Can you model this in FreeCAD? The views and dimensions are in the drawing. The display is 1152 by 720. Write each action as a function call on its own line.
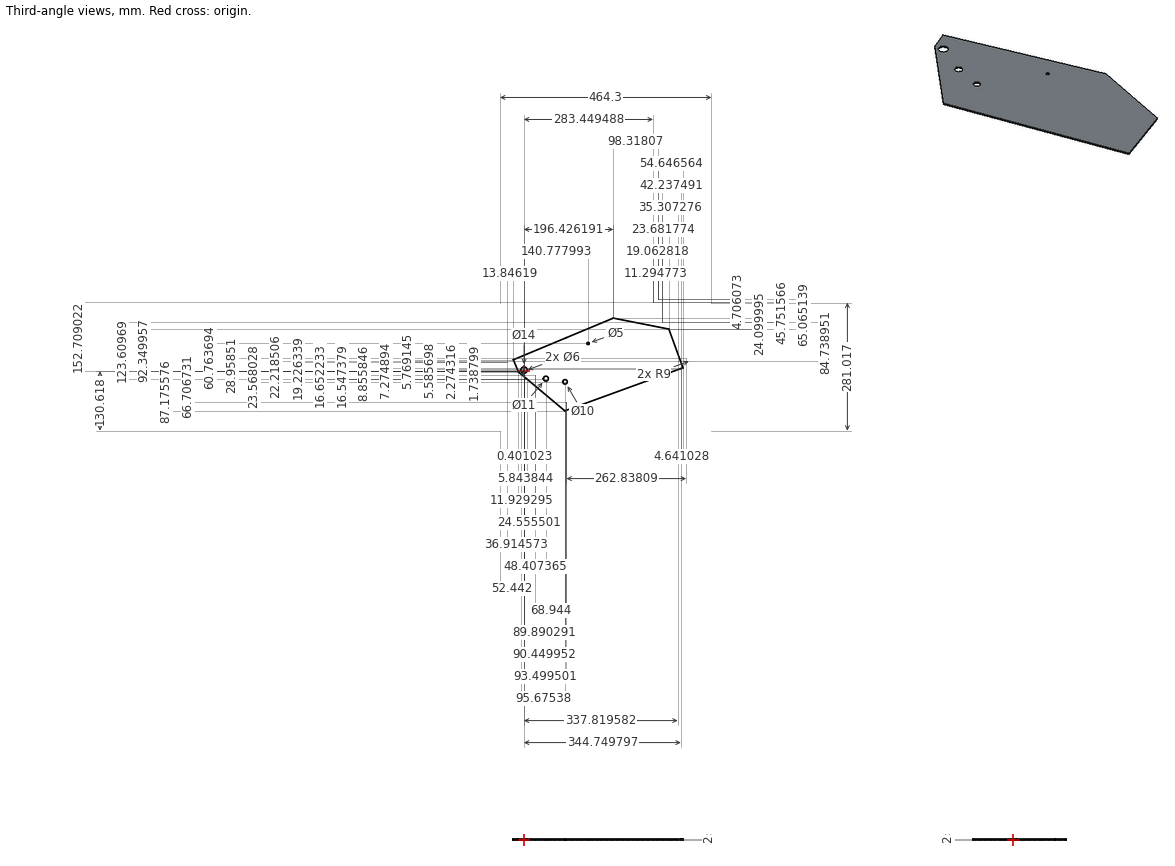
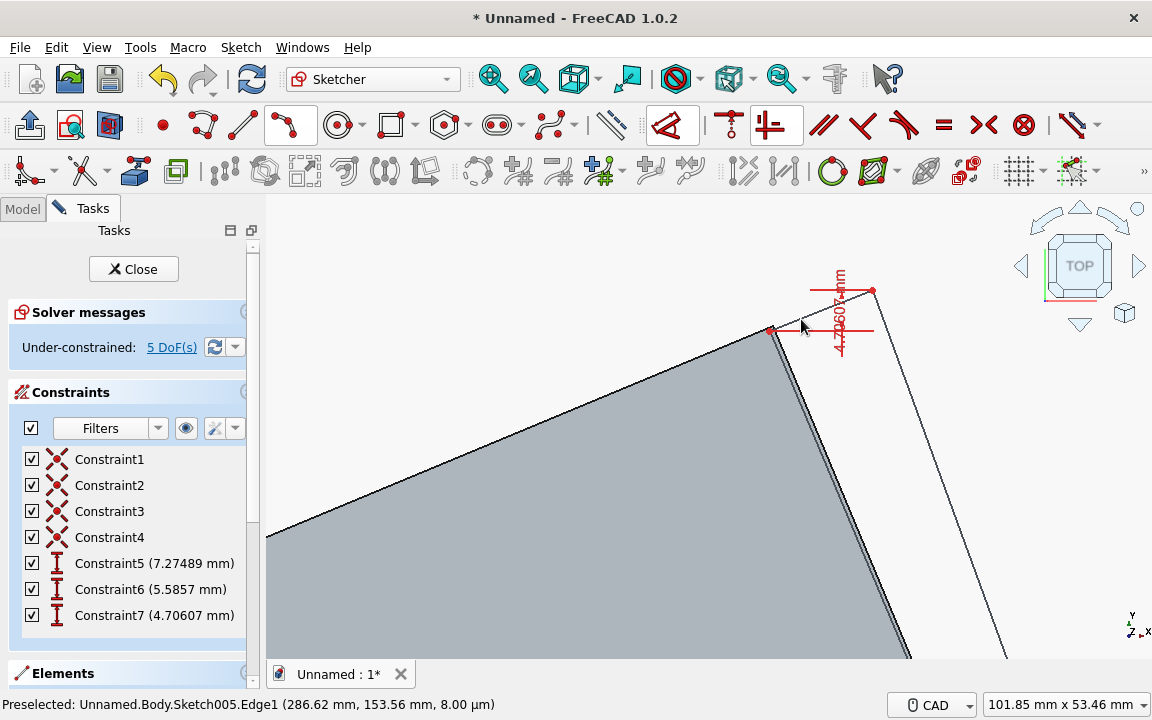
scroll(802, 319, down, 9)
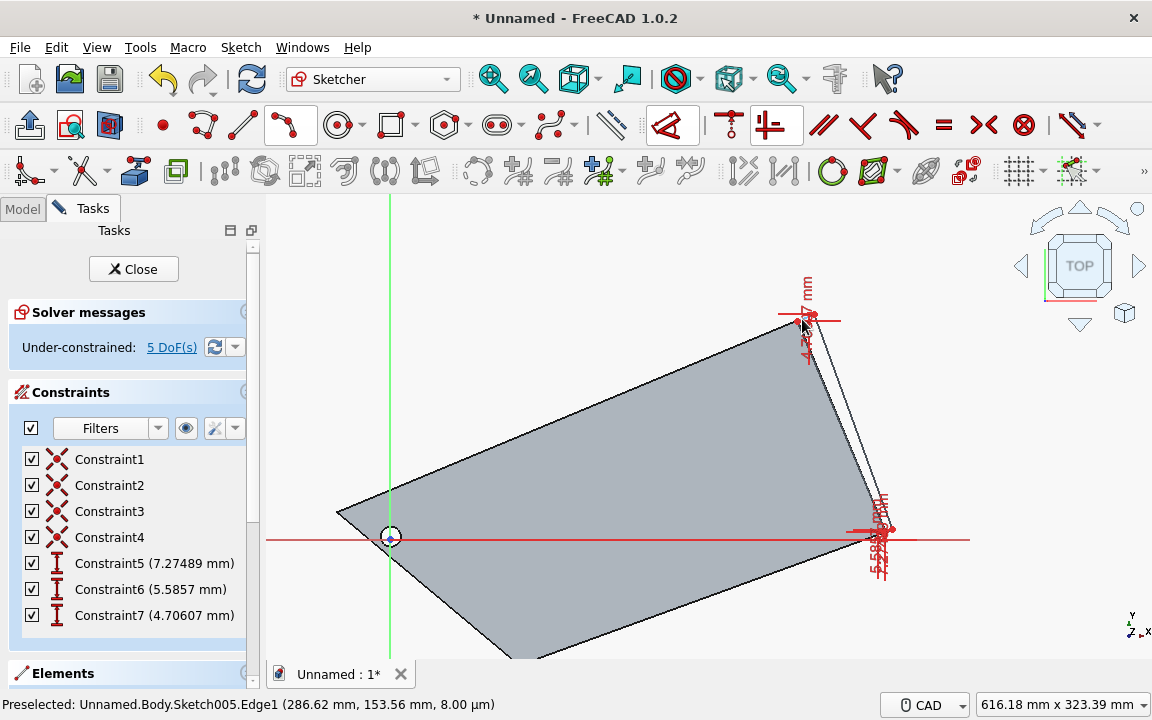
scroll(890, 530, up, 10)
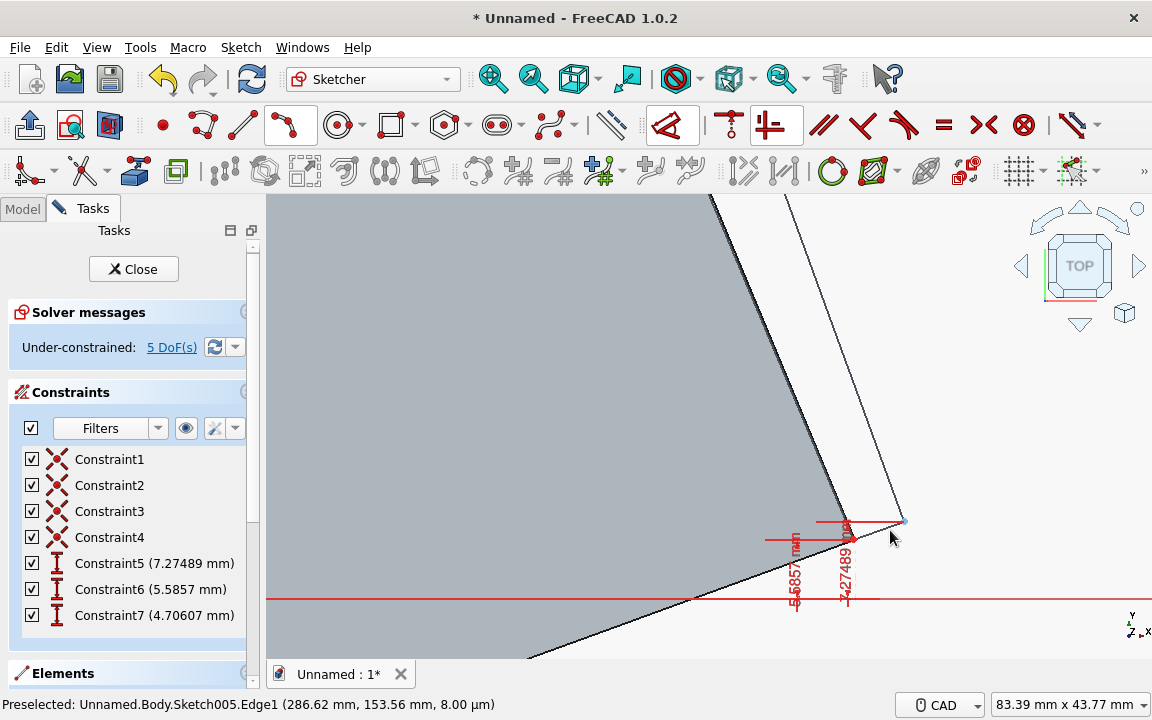
click(889, 527)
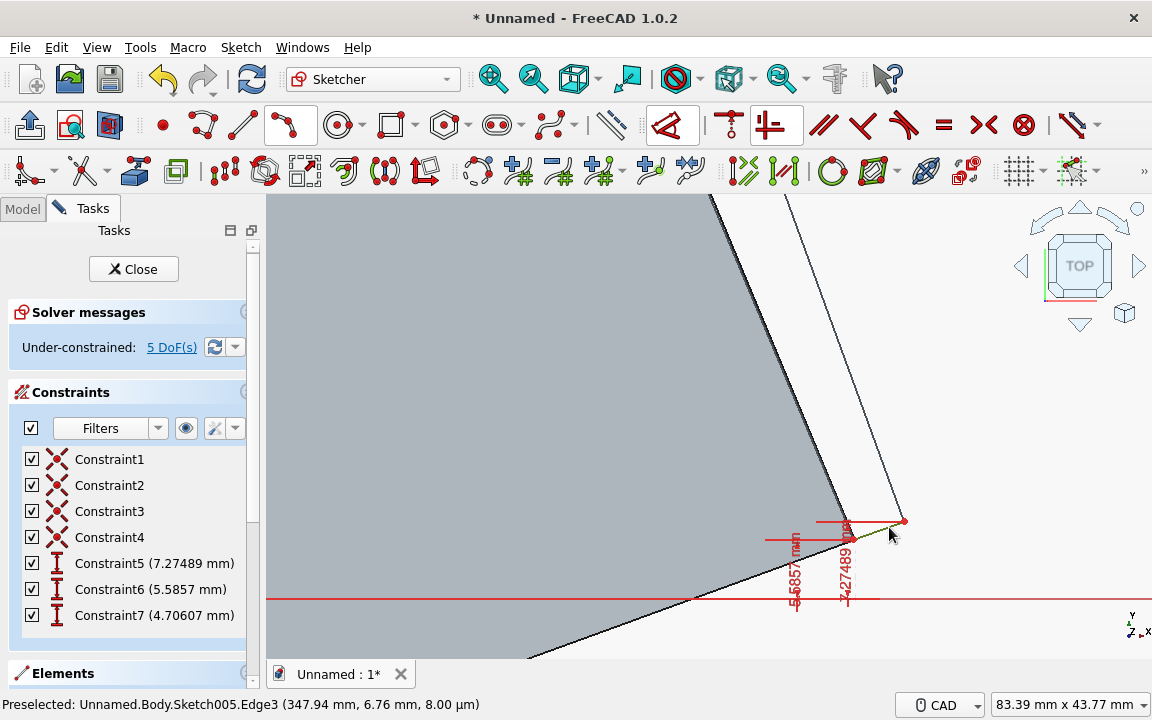
key(l)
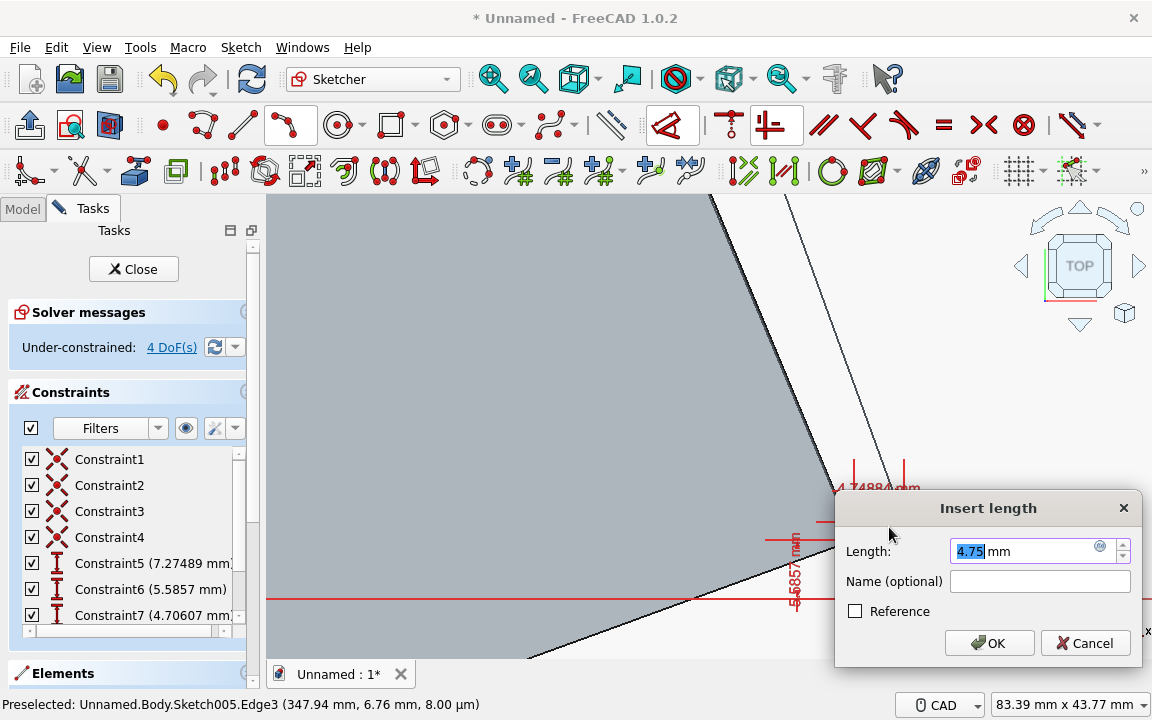
text(4.641028)
key(Return)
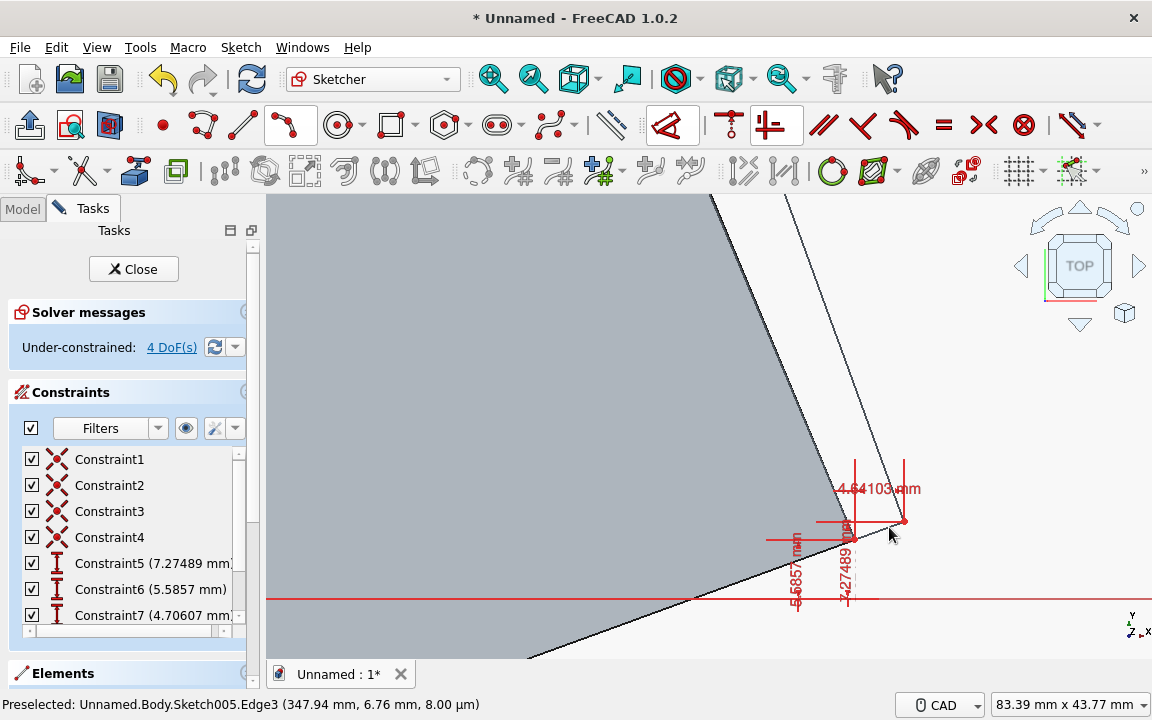
scroll(890, 530, down, 10)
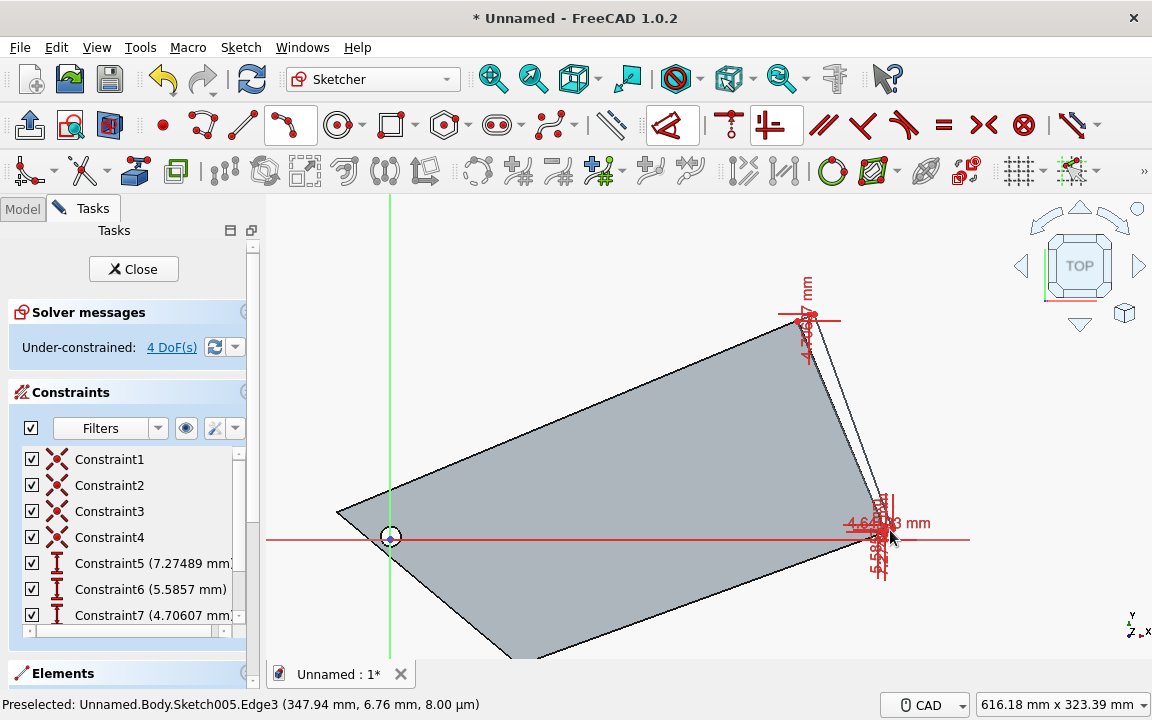
scroll(802, 319, up, 5)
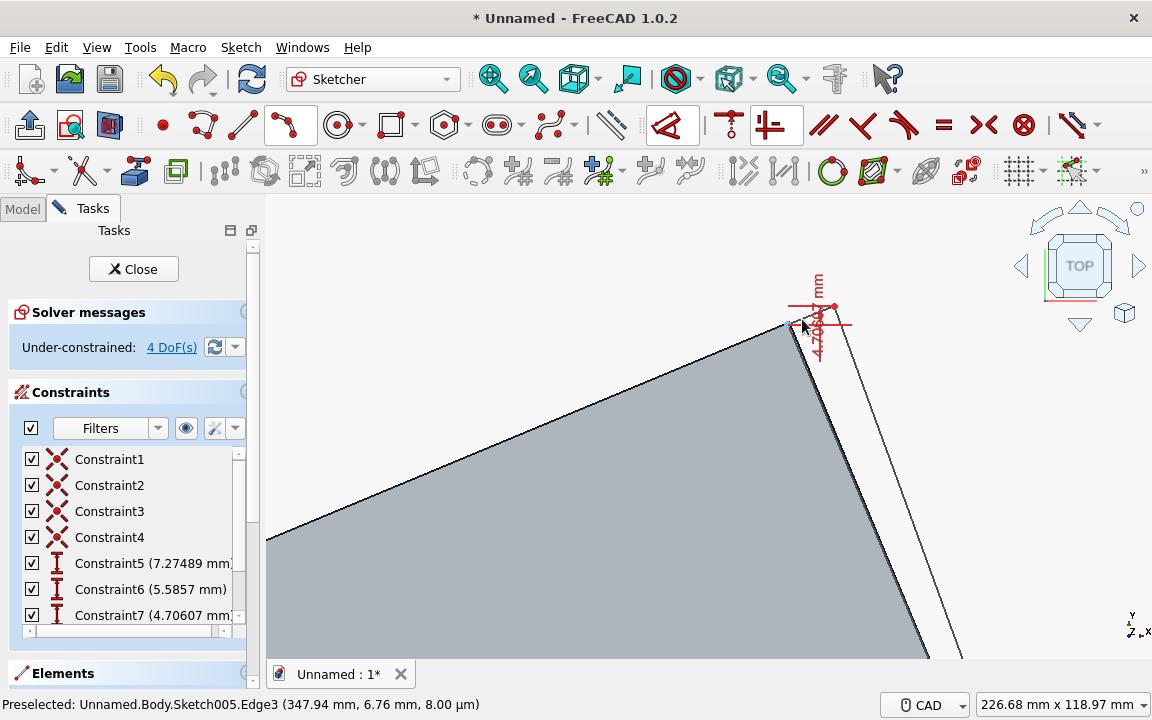
click(802, 319)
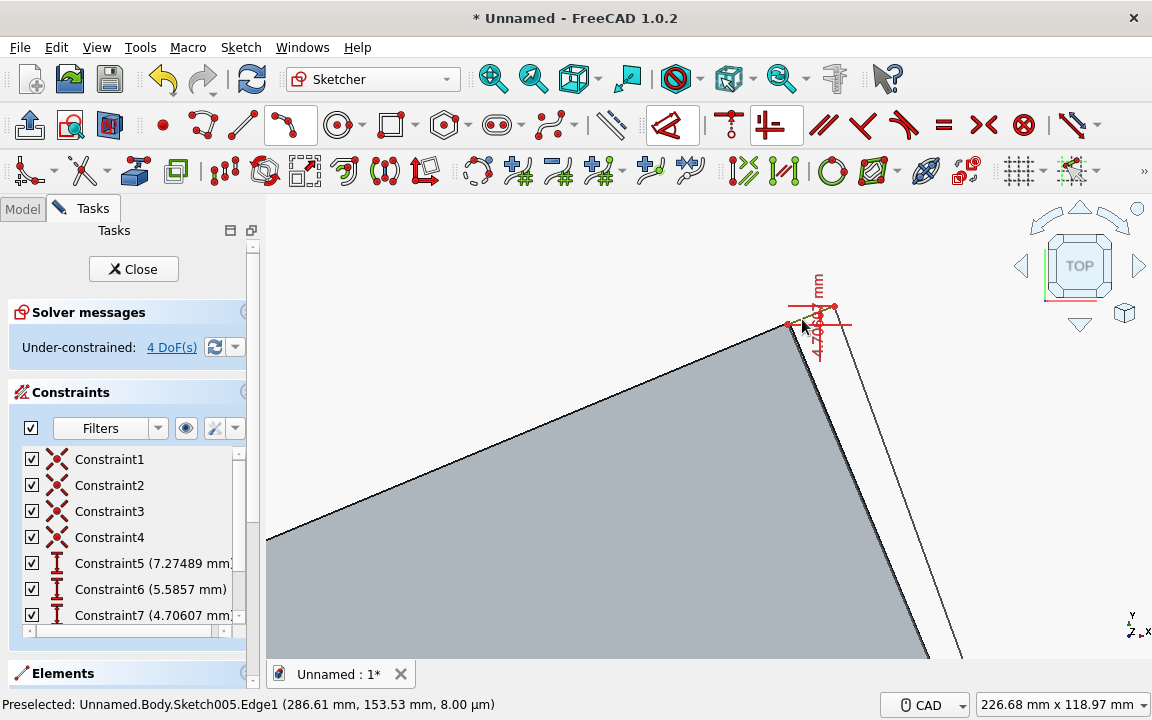
click(694, 126)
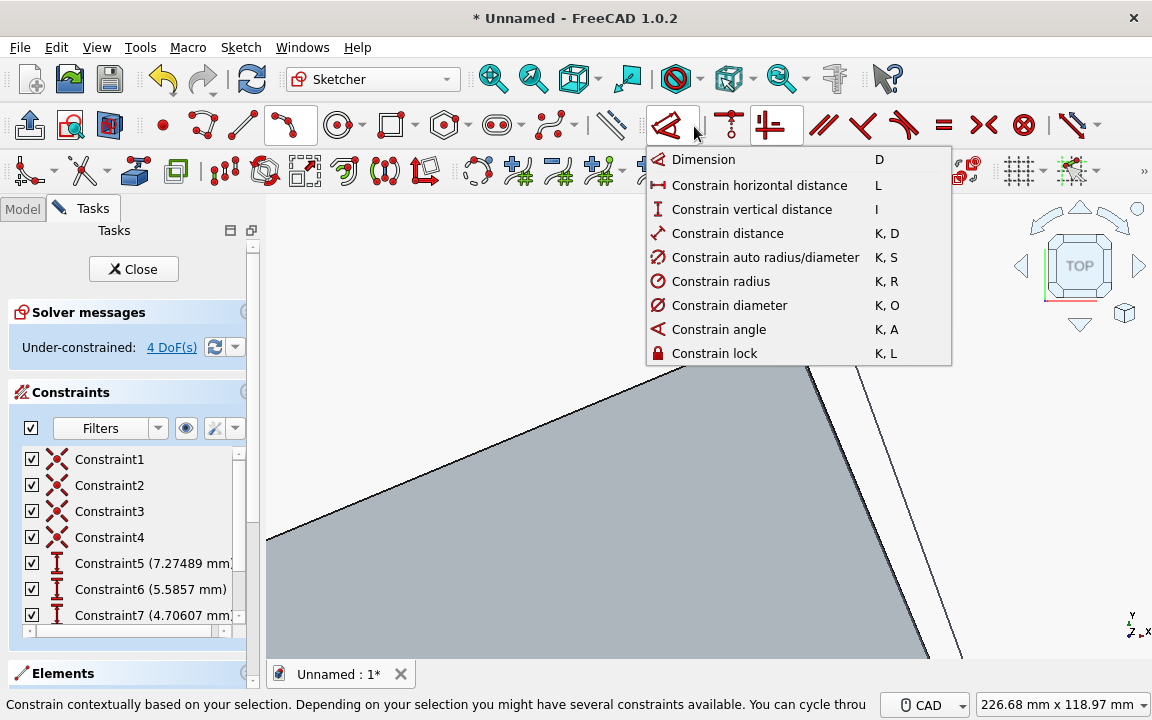
click(799, 185)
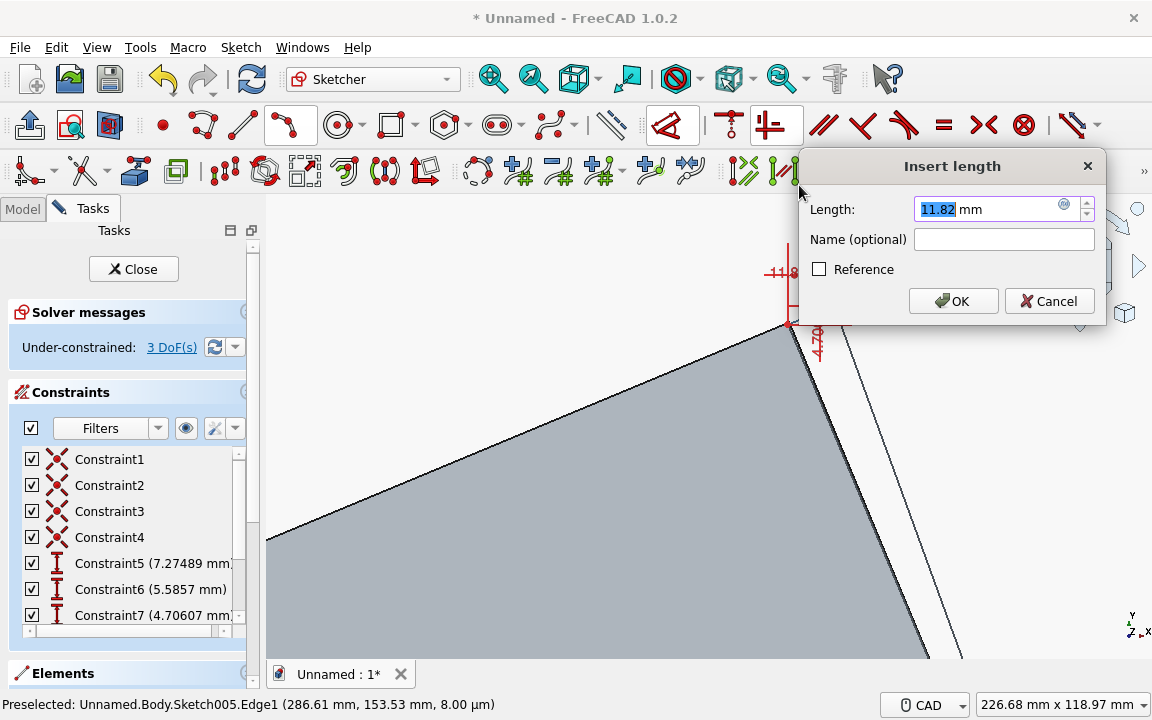
text(11.294773)
key(Return)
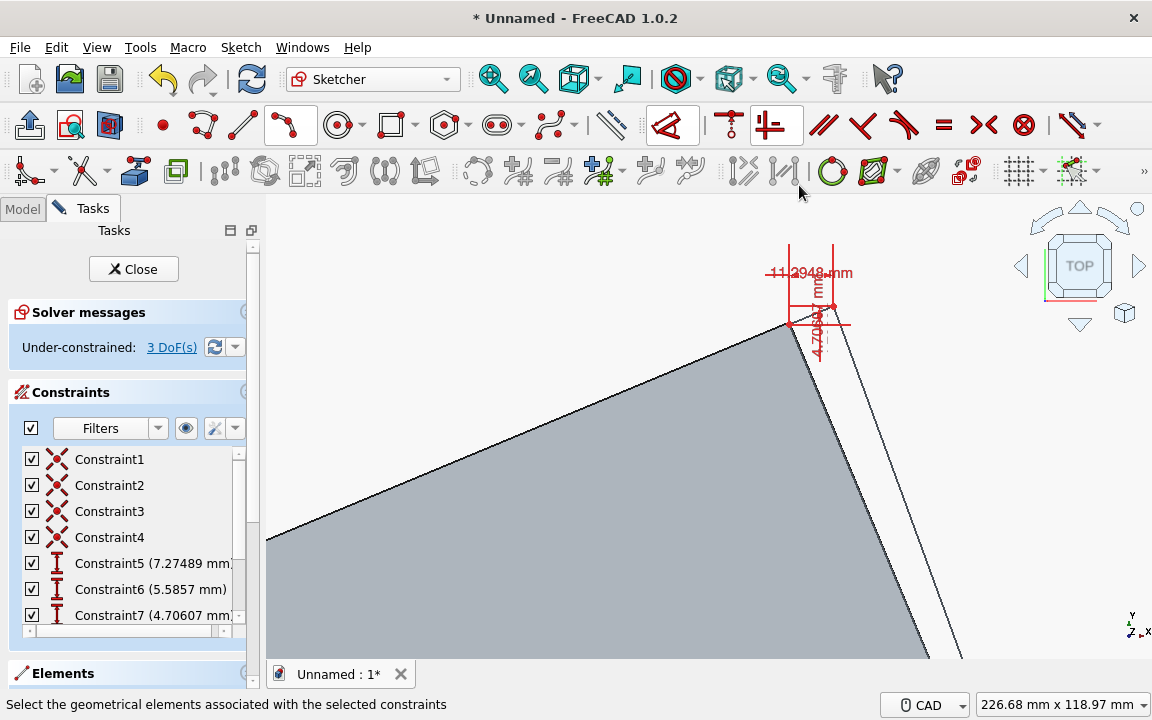
click(898, 482)